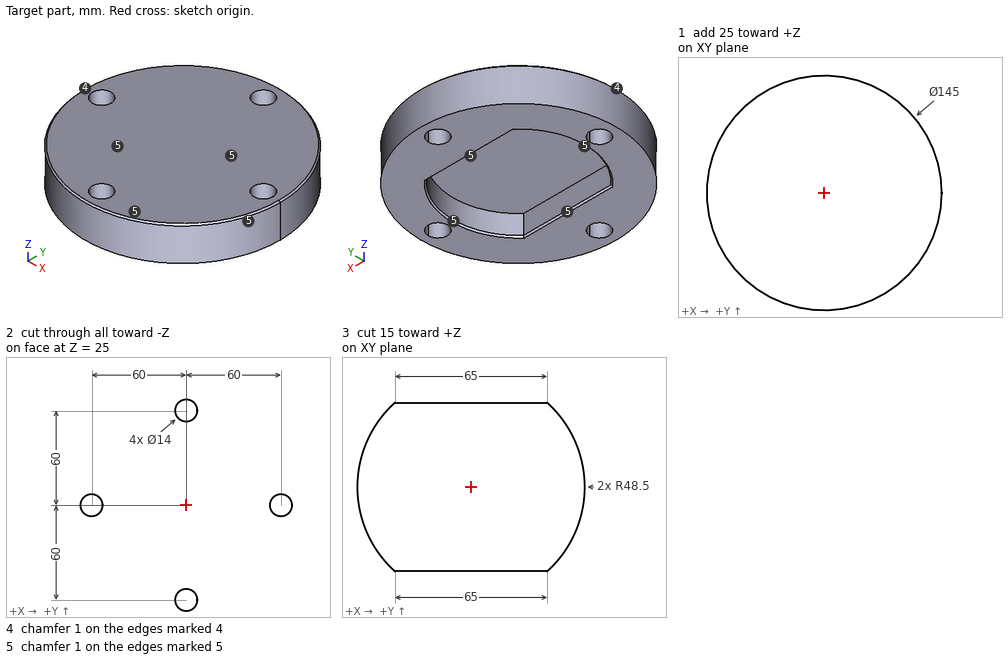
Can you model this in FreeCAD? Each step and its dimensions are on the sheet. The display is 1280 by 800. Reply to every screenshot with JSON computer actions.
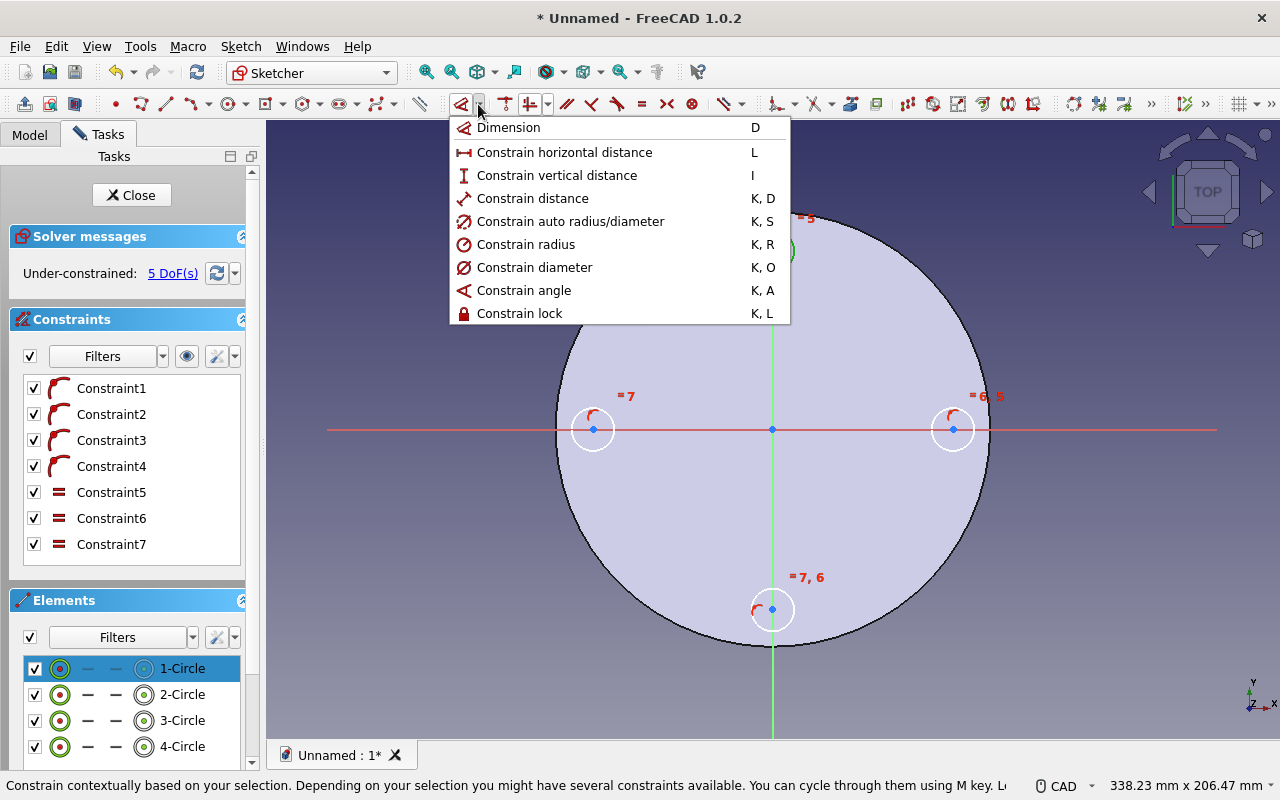
{"action": "left_click", "coordinate": [620, 268]}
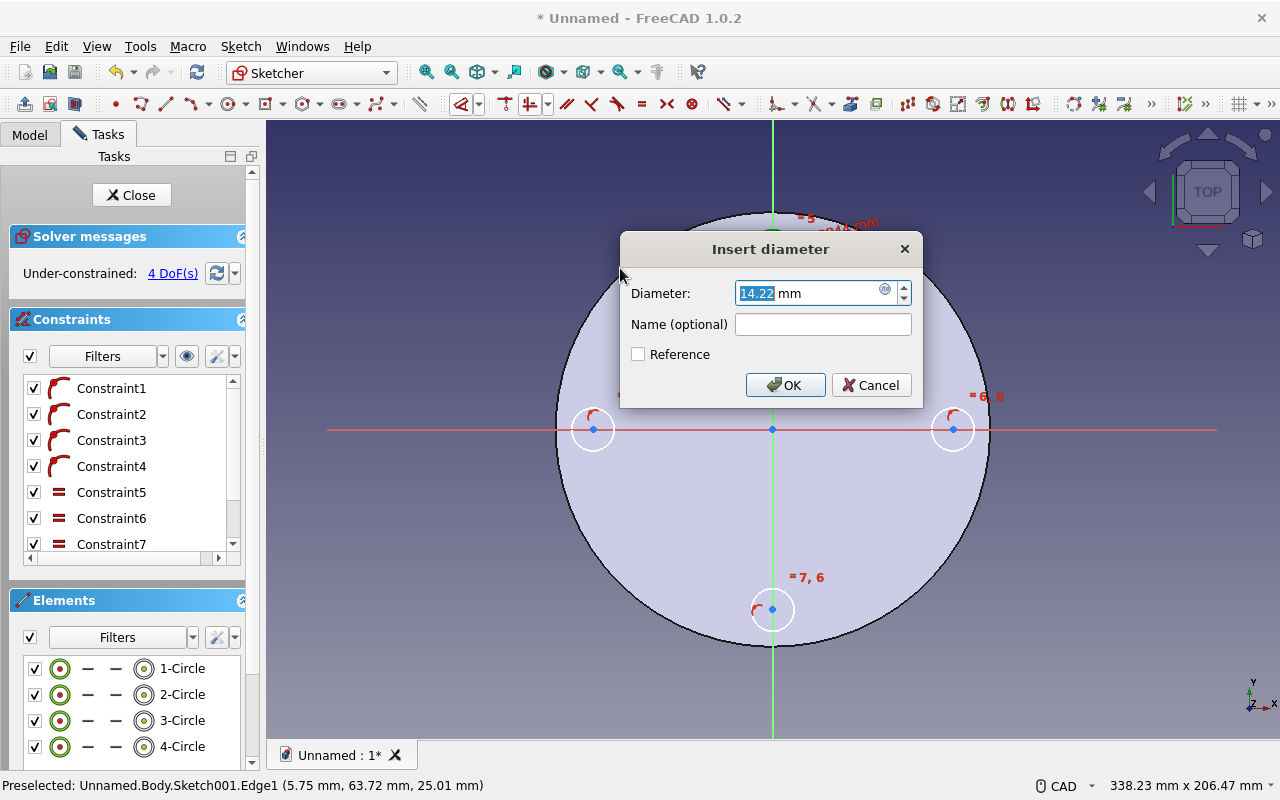
{"action": "type", "text": "14"}
{"action": "key", "text": "Return"}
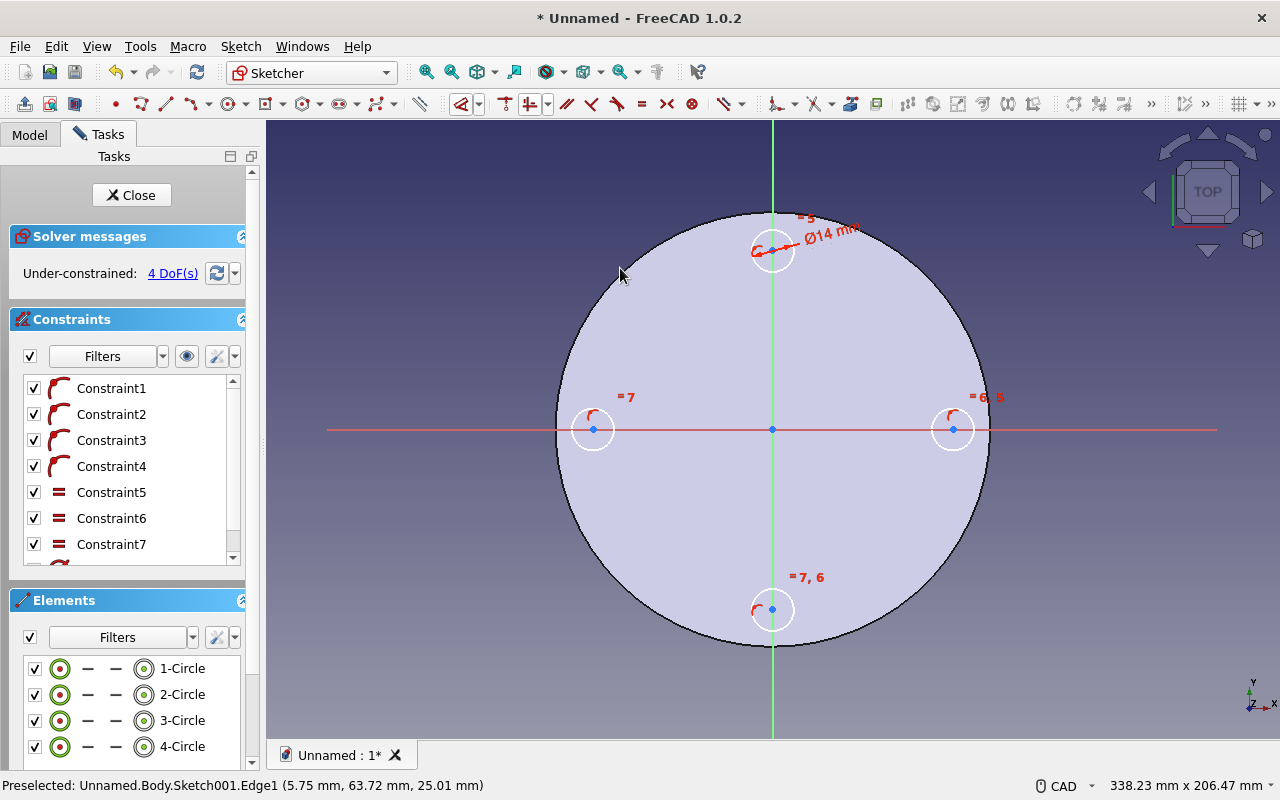
{"action": "left_click", "coordinate": [773, 251]}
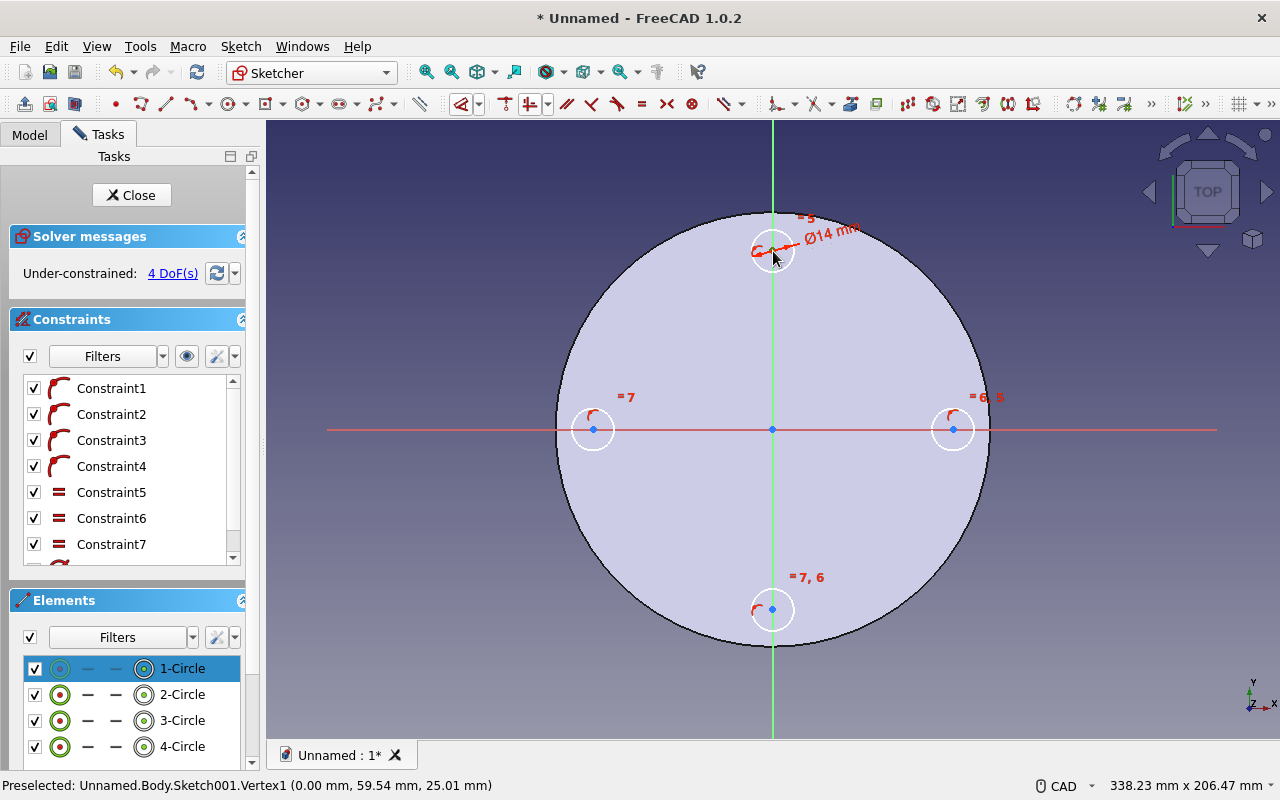
{"action": "left_click", "coordinate": [478, 104]}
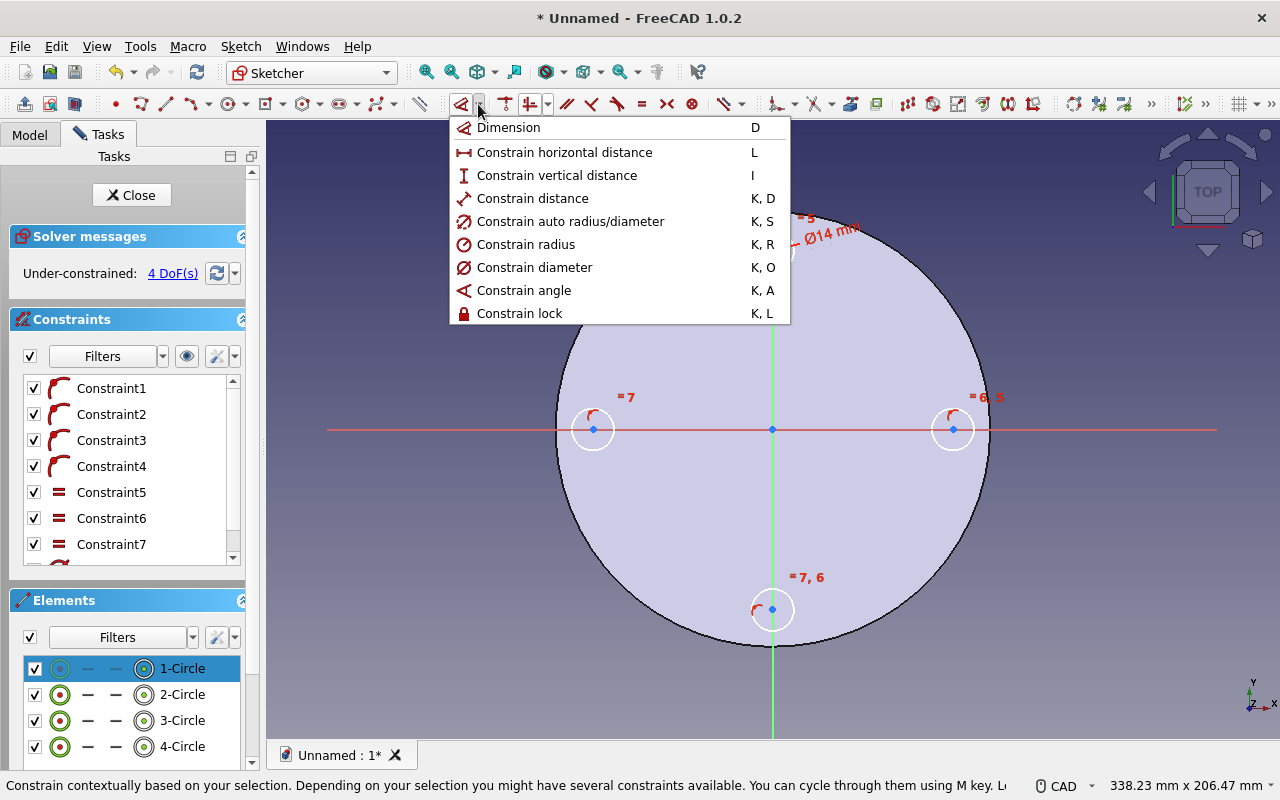
{"action": "left_click", "coordinate": [620, 176]}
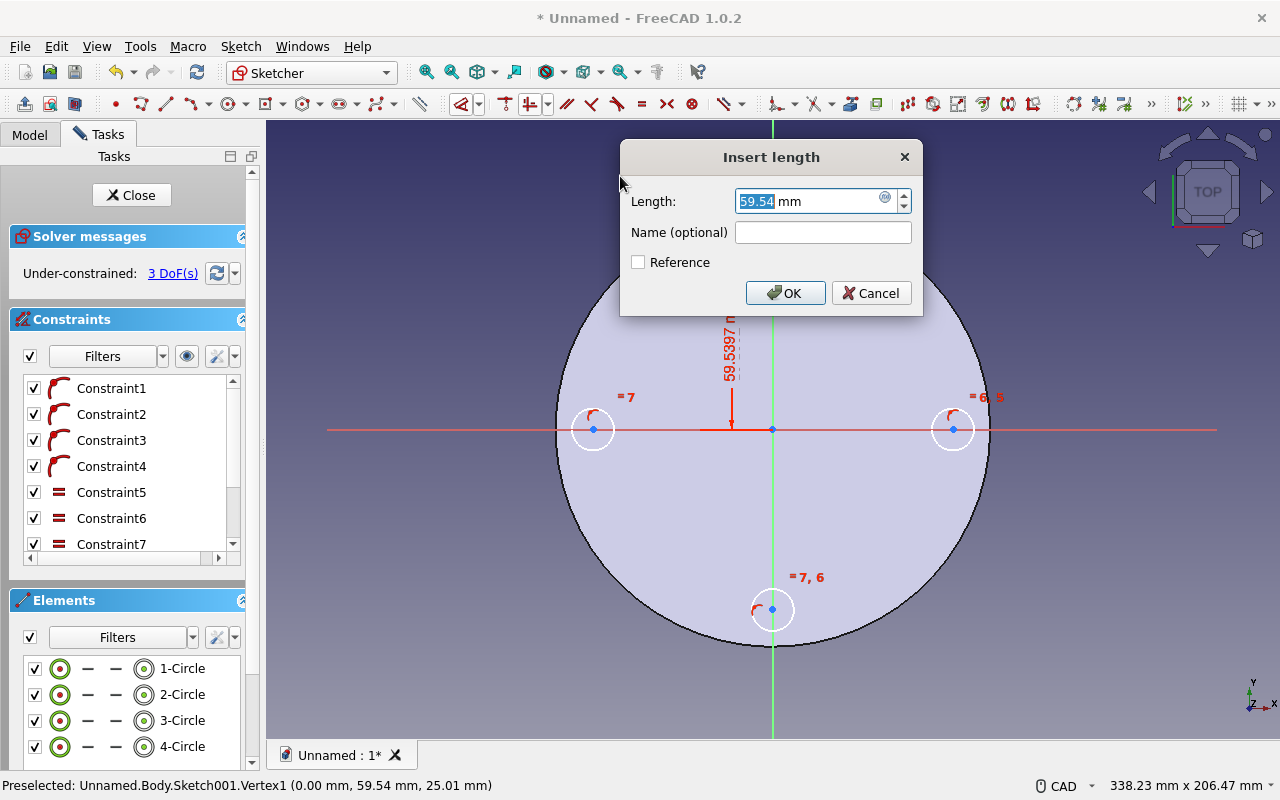
{"action": "type", "text": "60"}
{"action": "key", "text": "Return"}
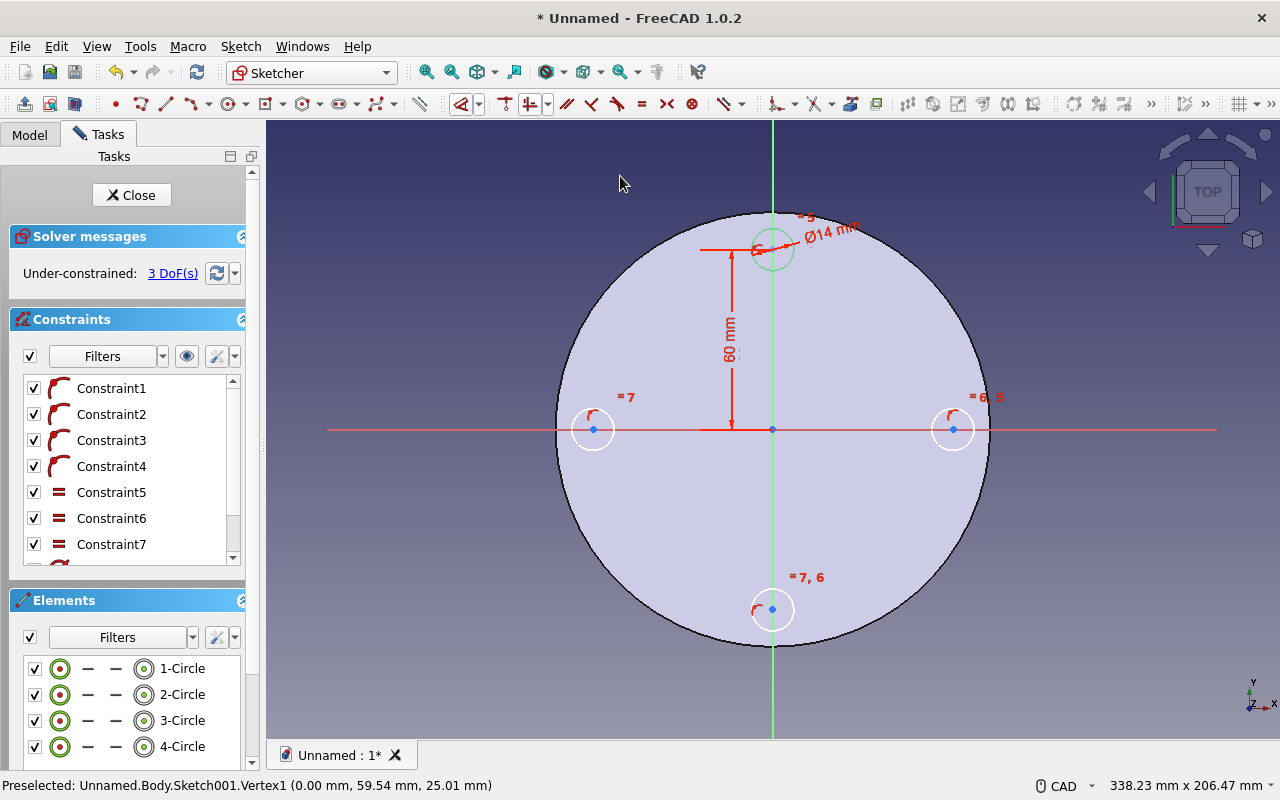
{"action": "left_click", "coordinate": [953, 430]}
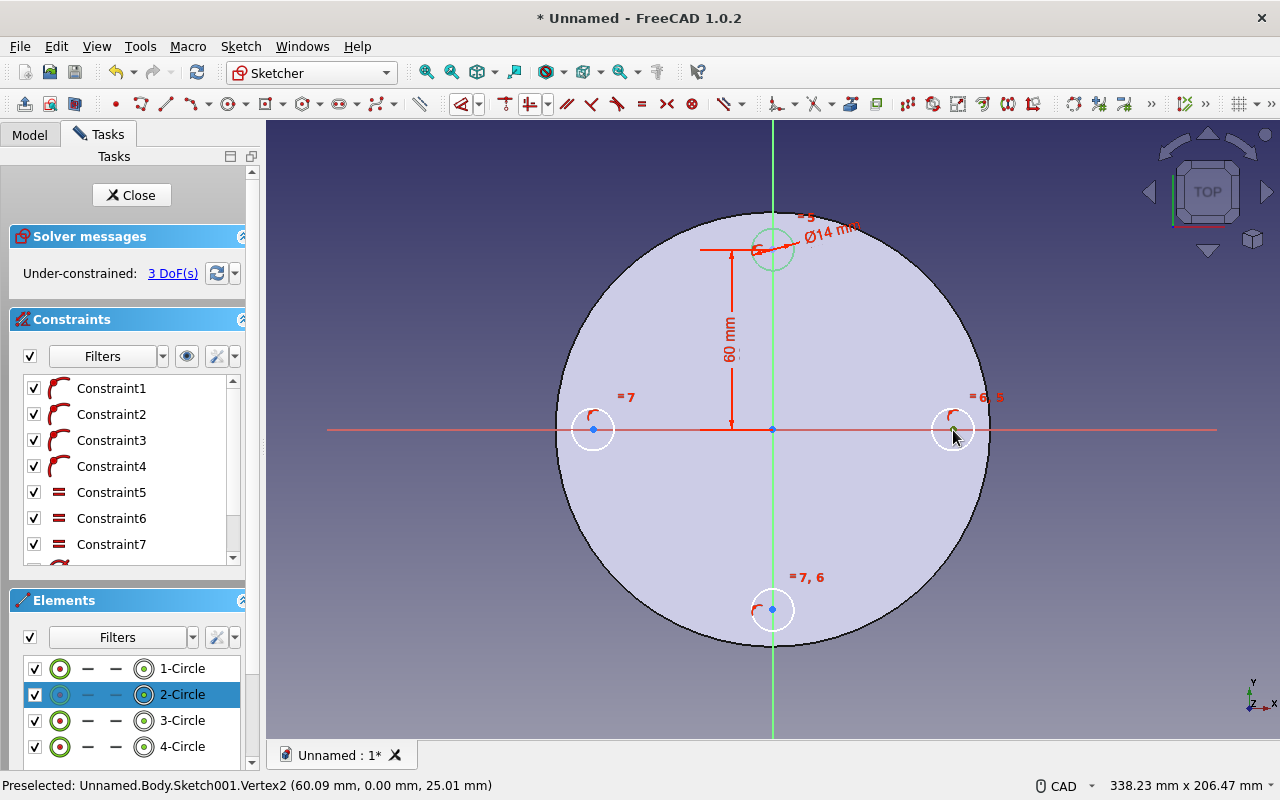
{"action": "left_click", "coordinate": [478, 104]}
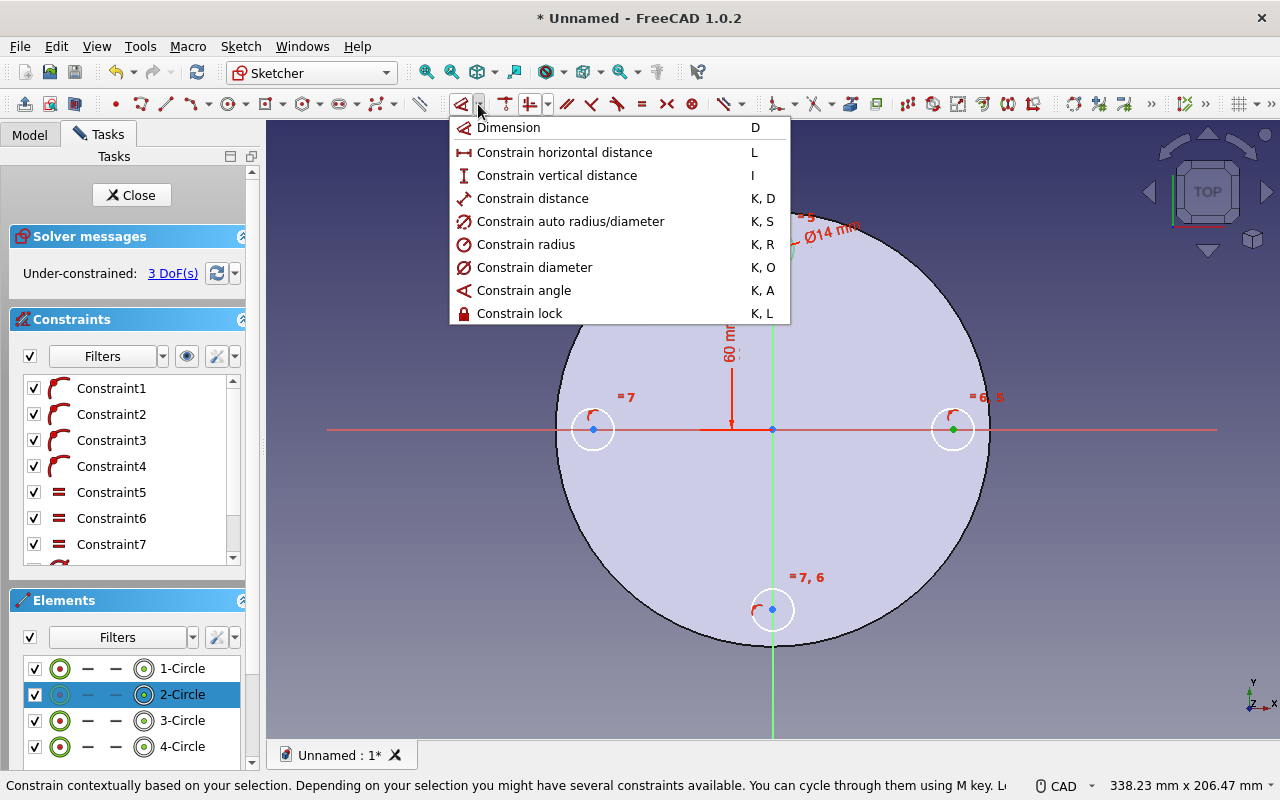
{"action": "left_click", "coordinate": [620, 152]}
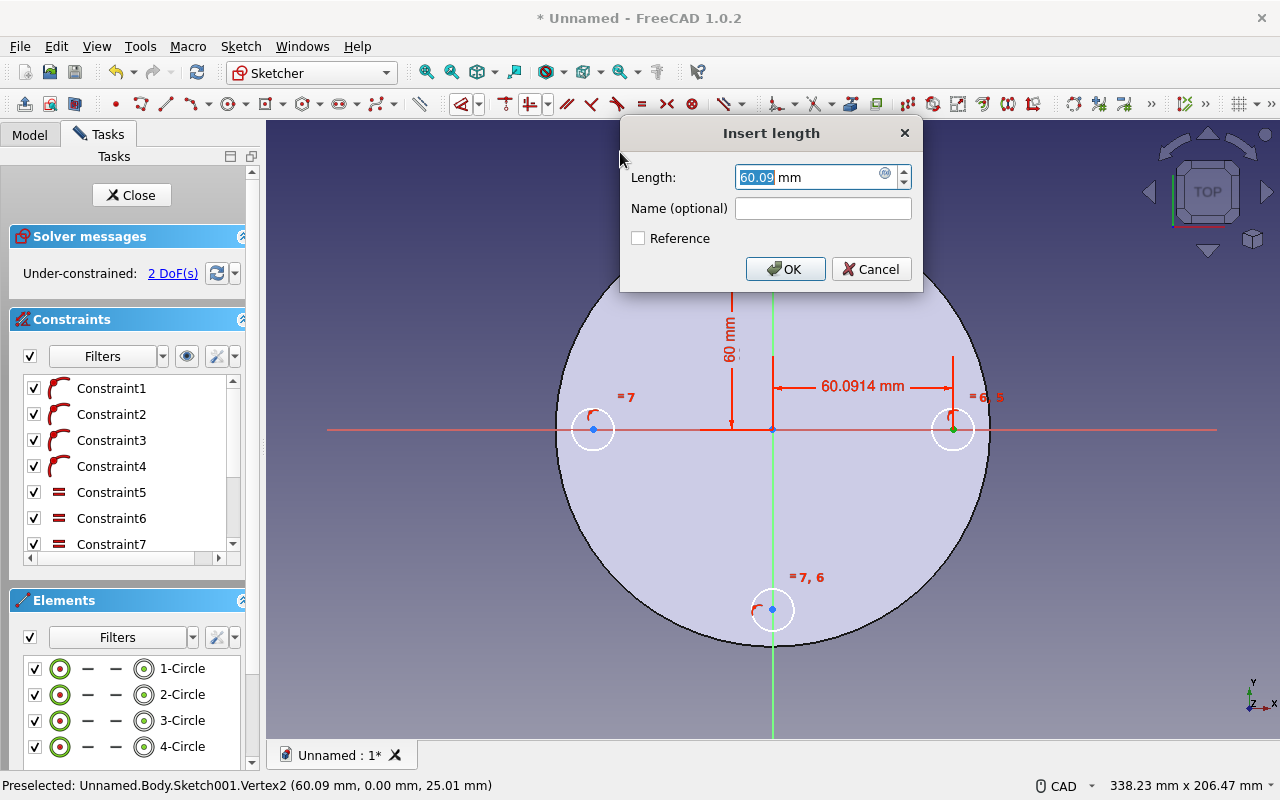
{"action": "type", "text": "60"}
{"action": "key", "text": "Return"}